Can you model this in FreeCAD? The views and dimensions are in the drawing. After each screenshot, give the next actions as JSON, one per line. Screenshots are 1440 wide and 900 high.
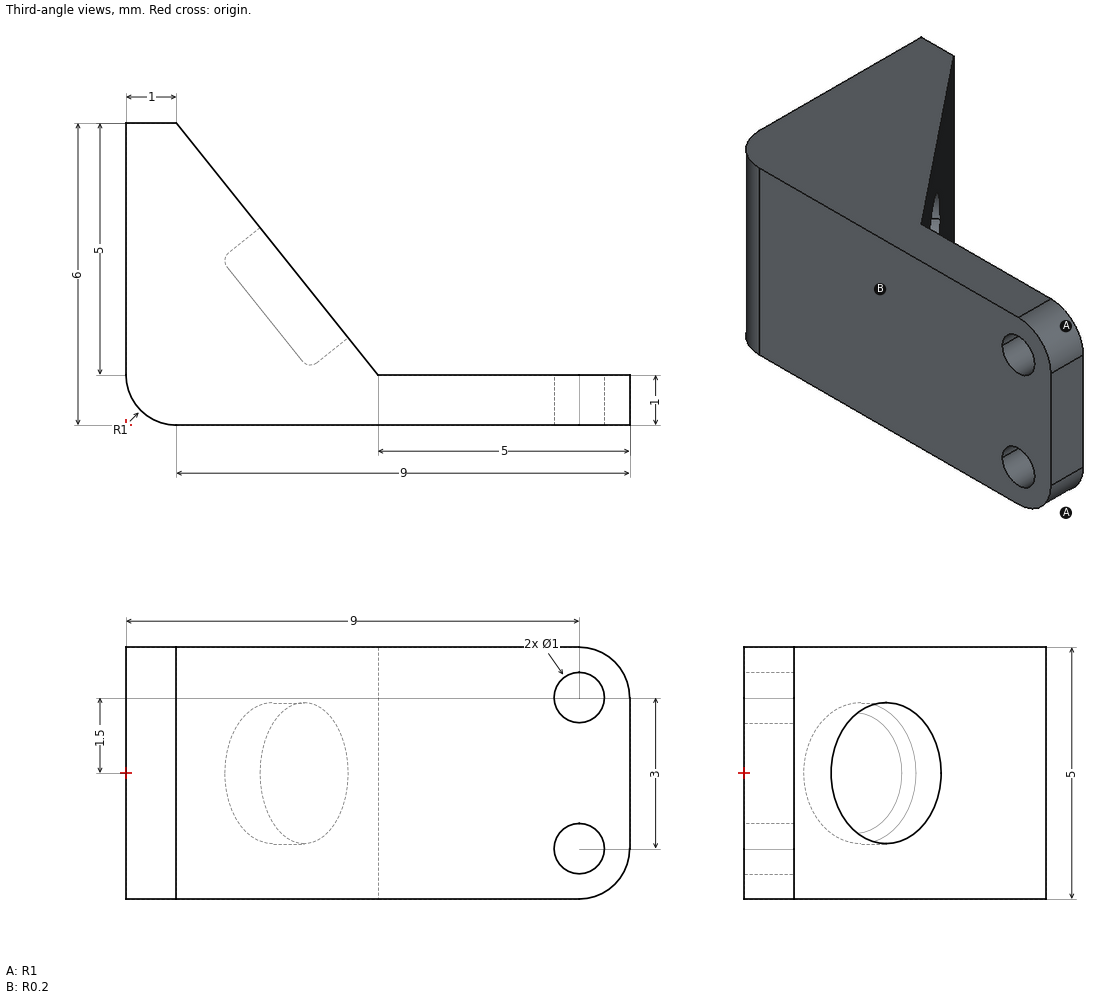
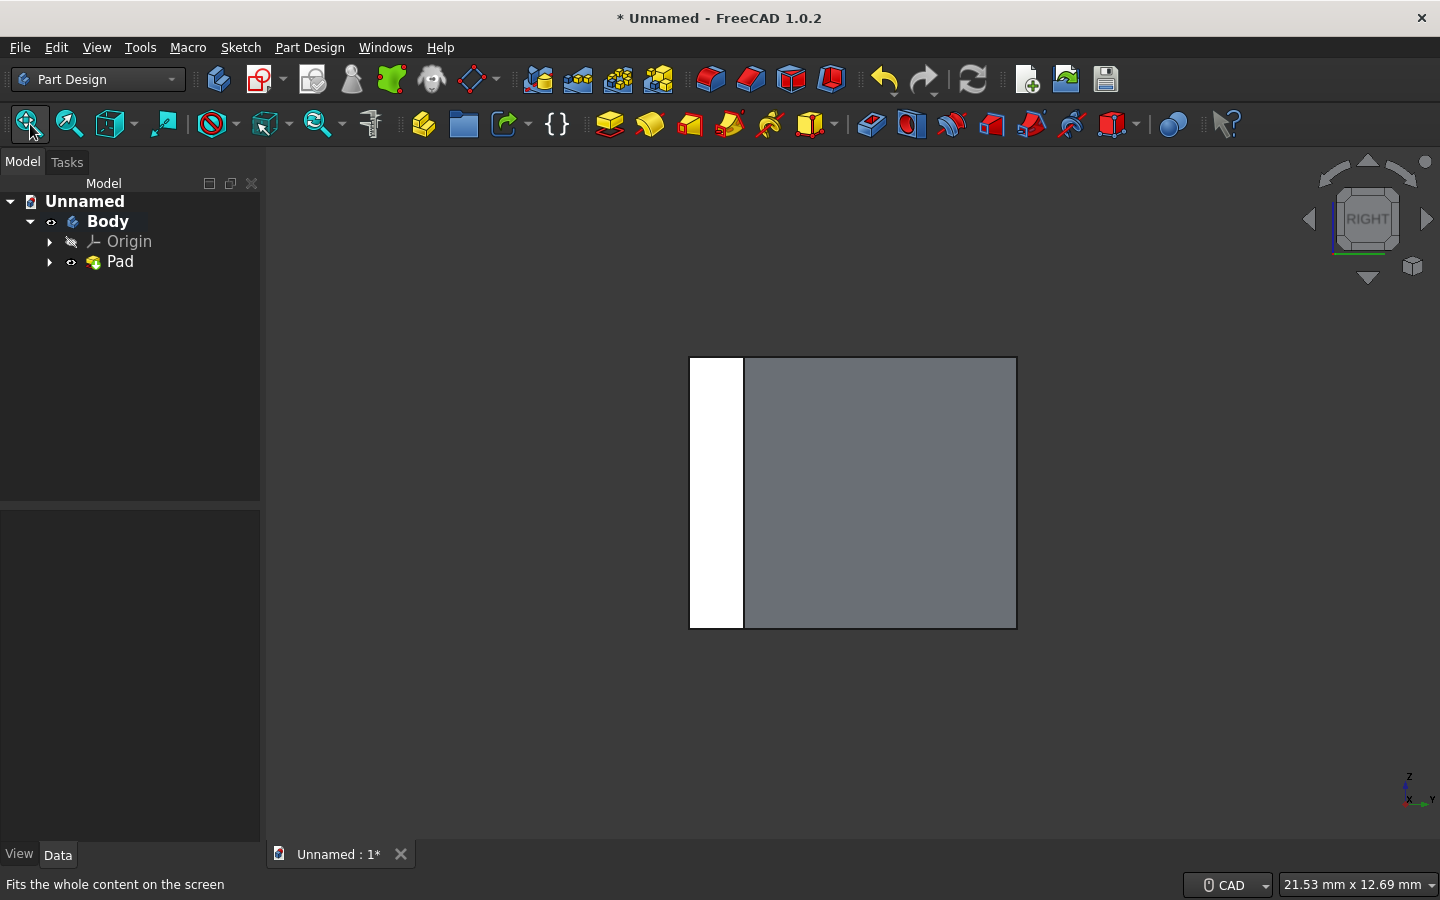
{"action": "left_click", "coordinate": [880, 492]}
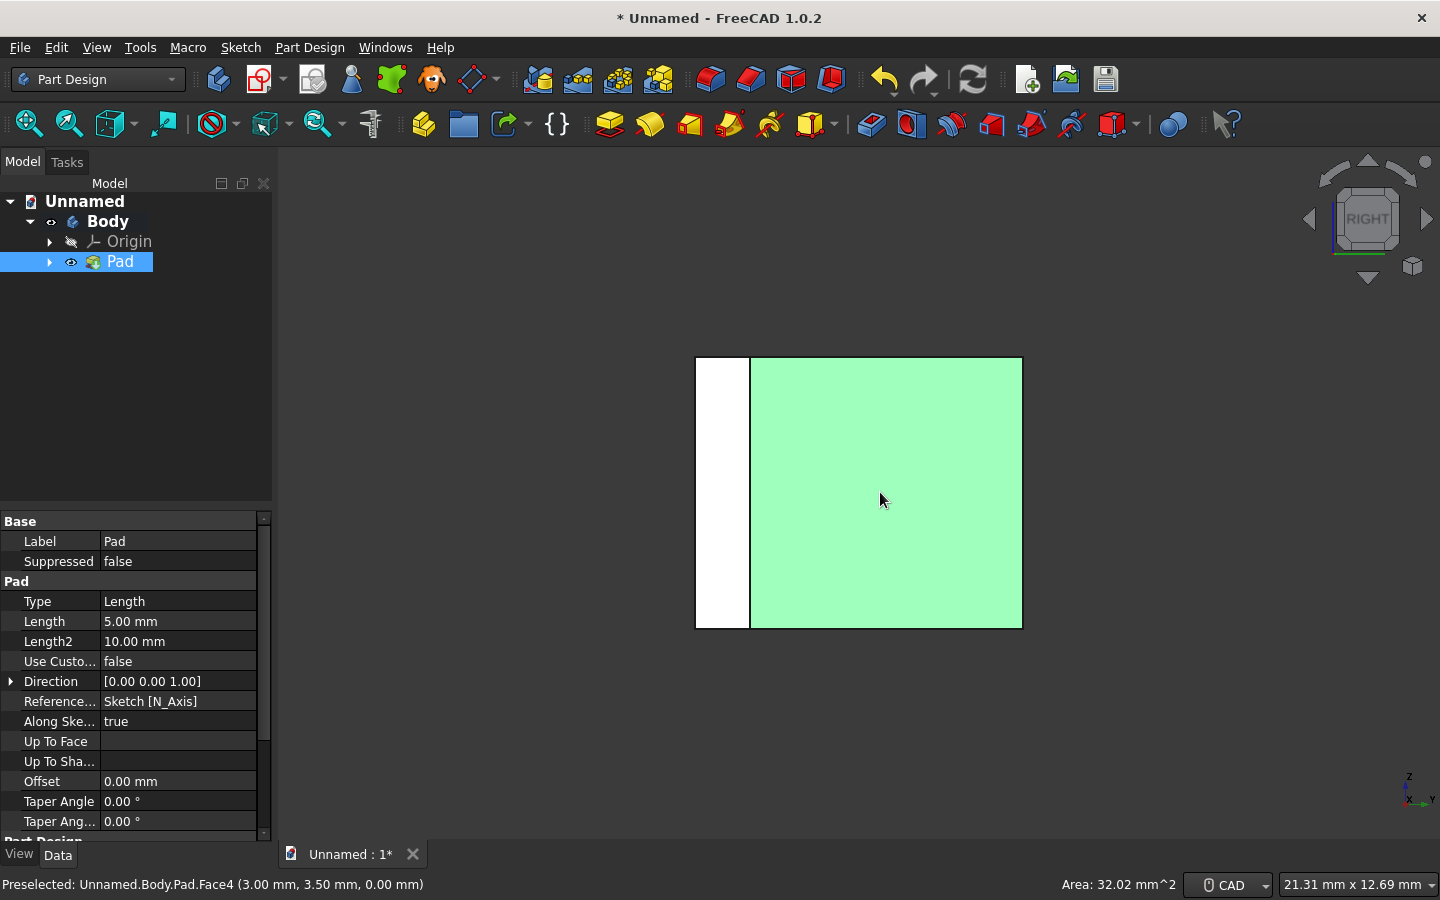
{"action": "left_click", "coordinate": [260, 80]}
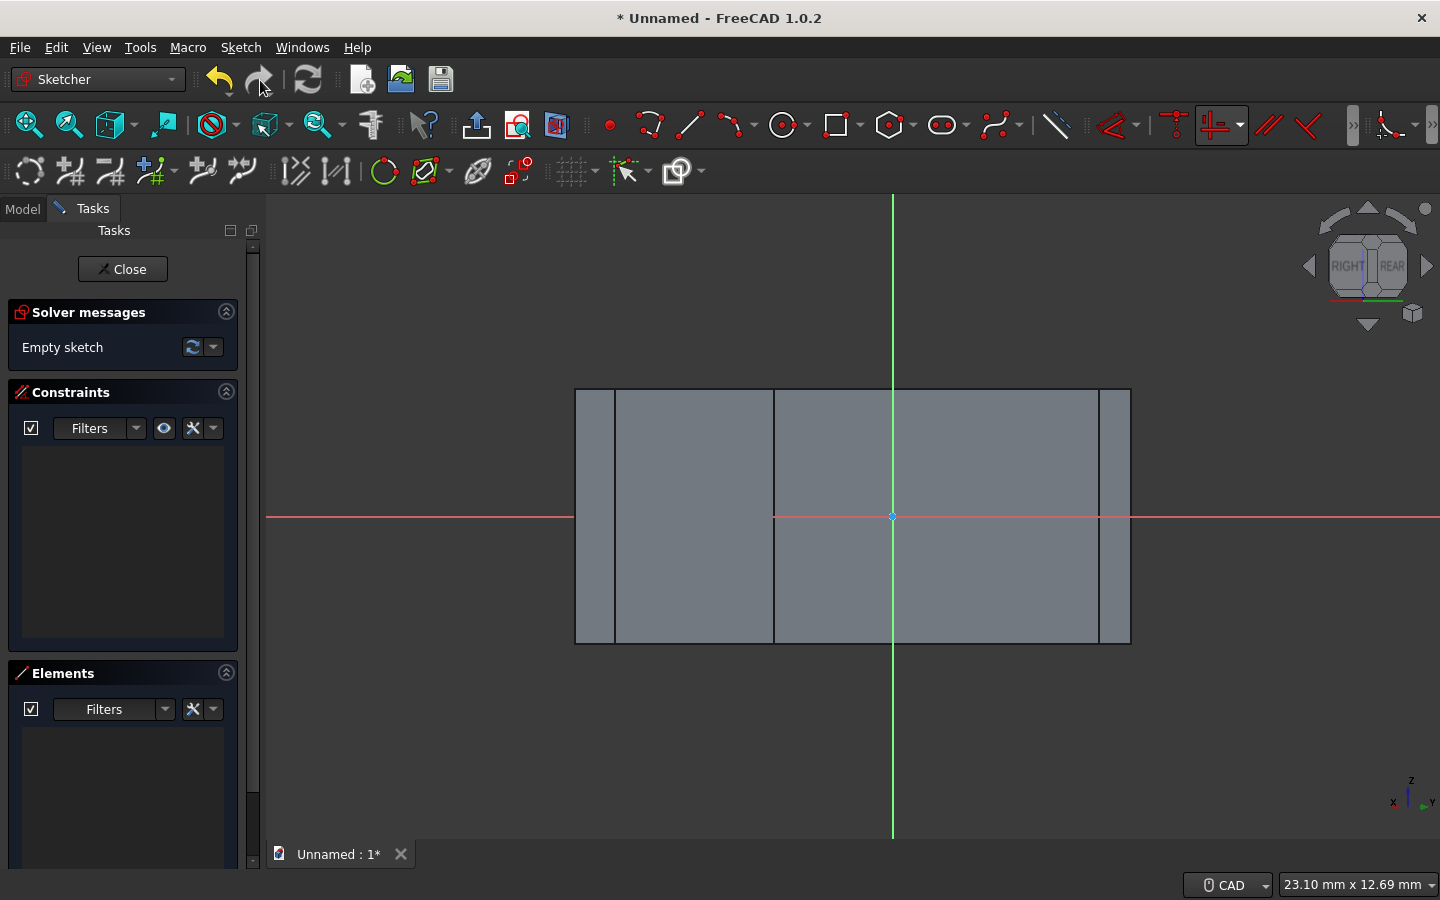
{"action": "scroll", "coordinate": [956, 516], "scroll_direction": "up", "scroll_amount": 5}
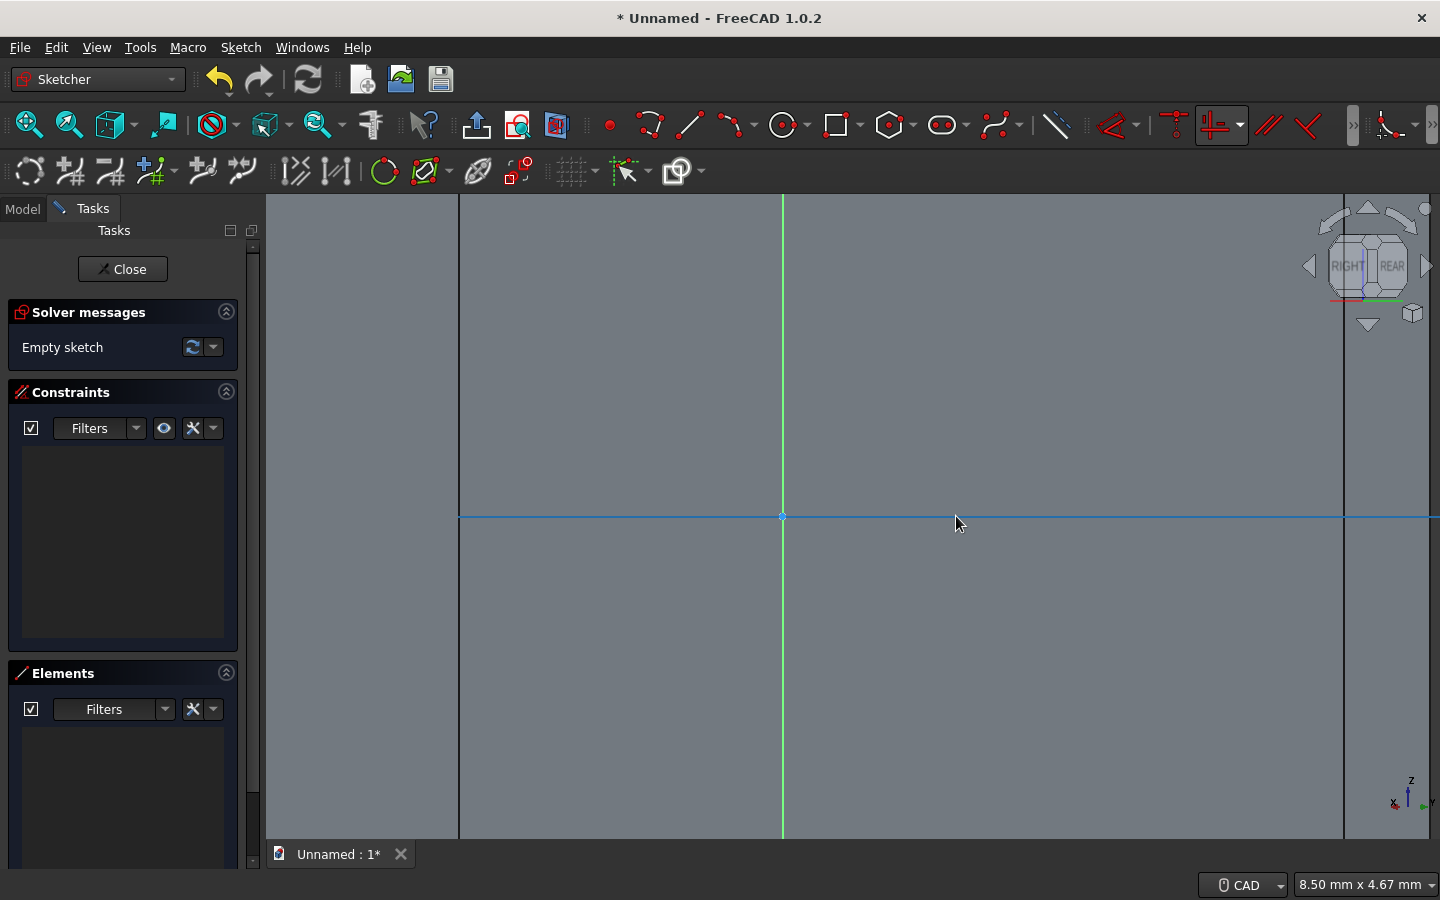
{"action": "left_click", "coordinate": [784, 126]}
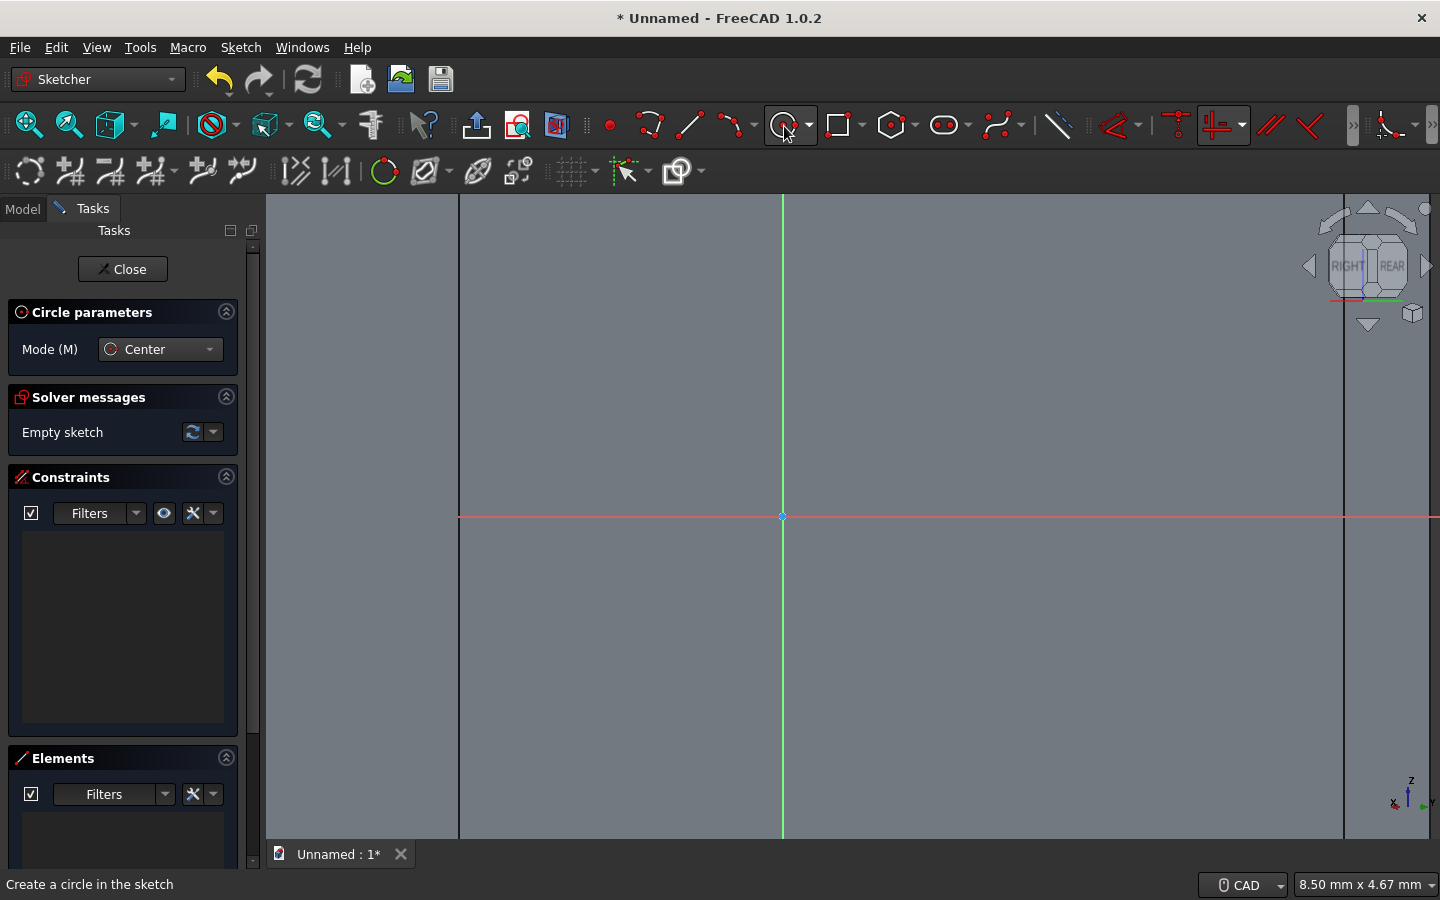
{"action": "left_click", "coordinate": [783, 516]}
{"action": "mouse_move", "coordinate": [920, 380]}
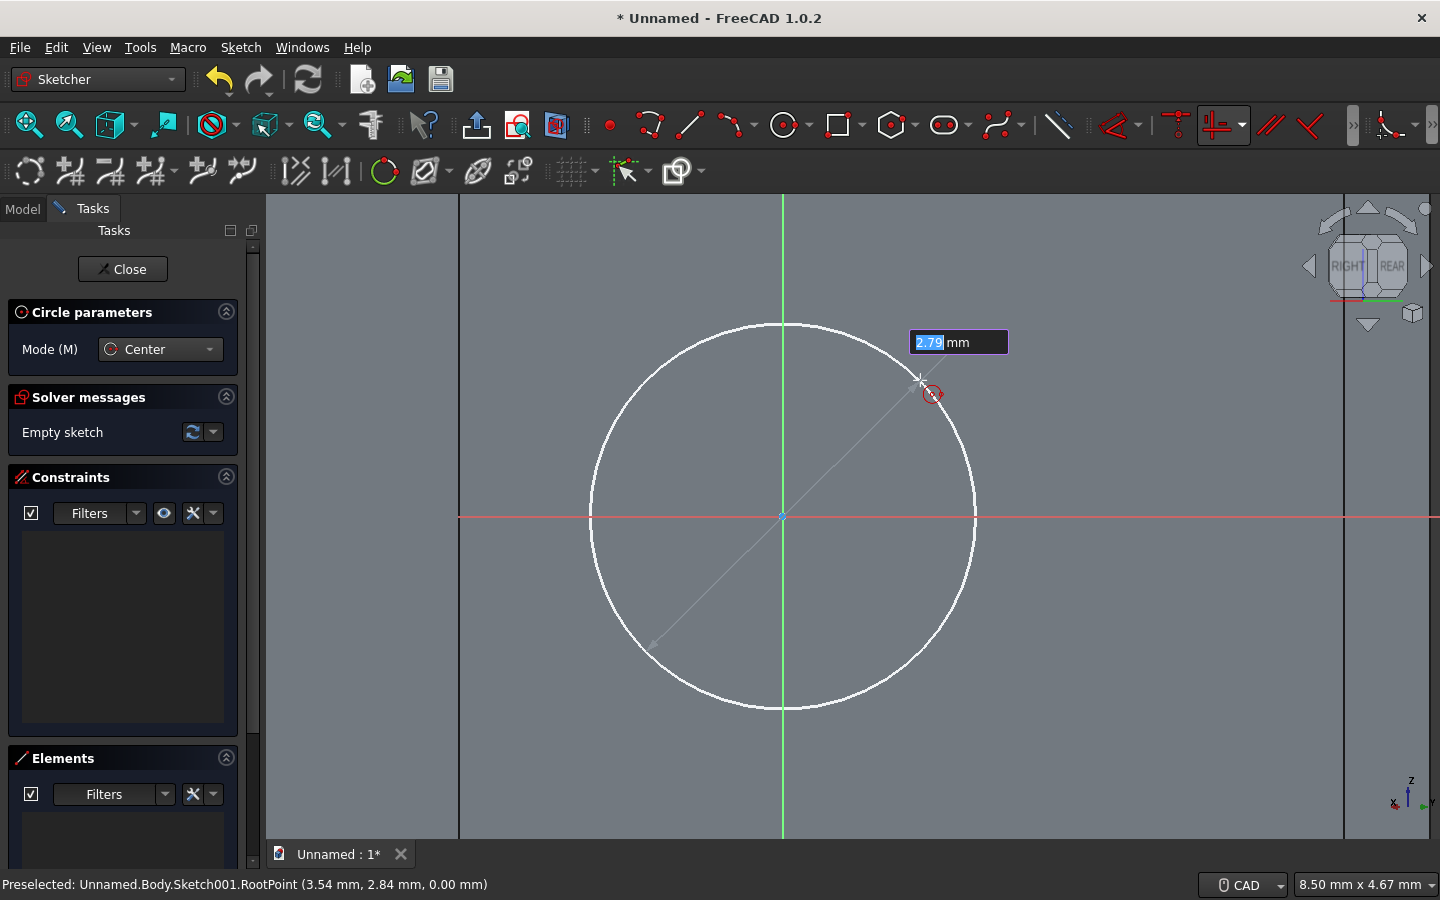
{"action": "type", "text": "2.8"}
{"action": "key", "text": "Return"}
{"action": "key", "text": "Escape"}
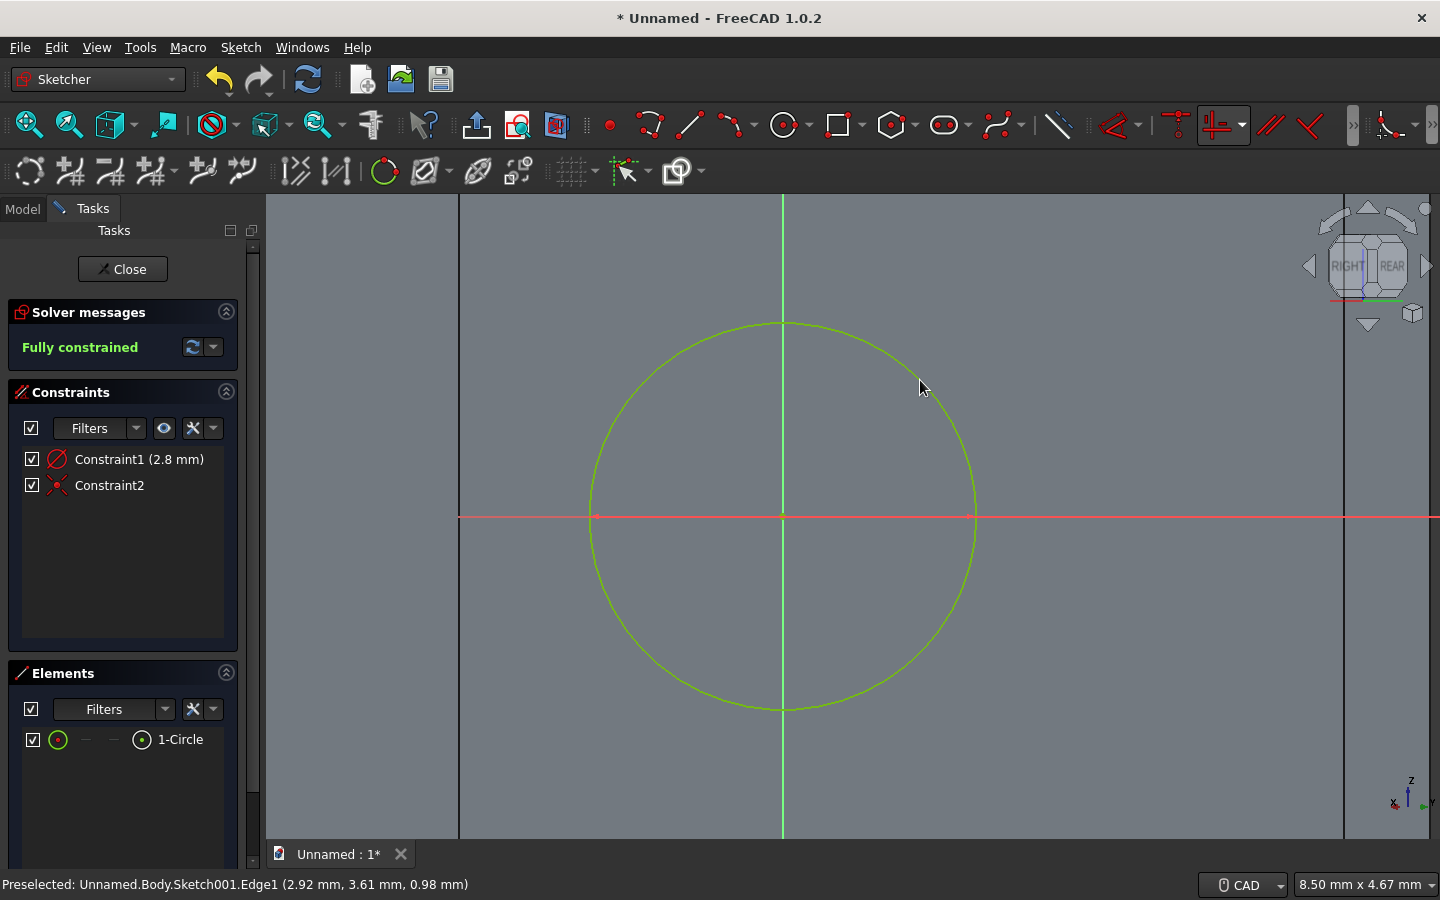
{"action": "left_click", "coordinate": [123, 269]}